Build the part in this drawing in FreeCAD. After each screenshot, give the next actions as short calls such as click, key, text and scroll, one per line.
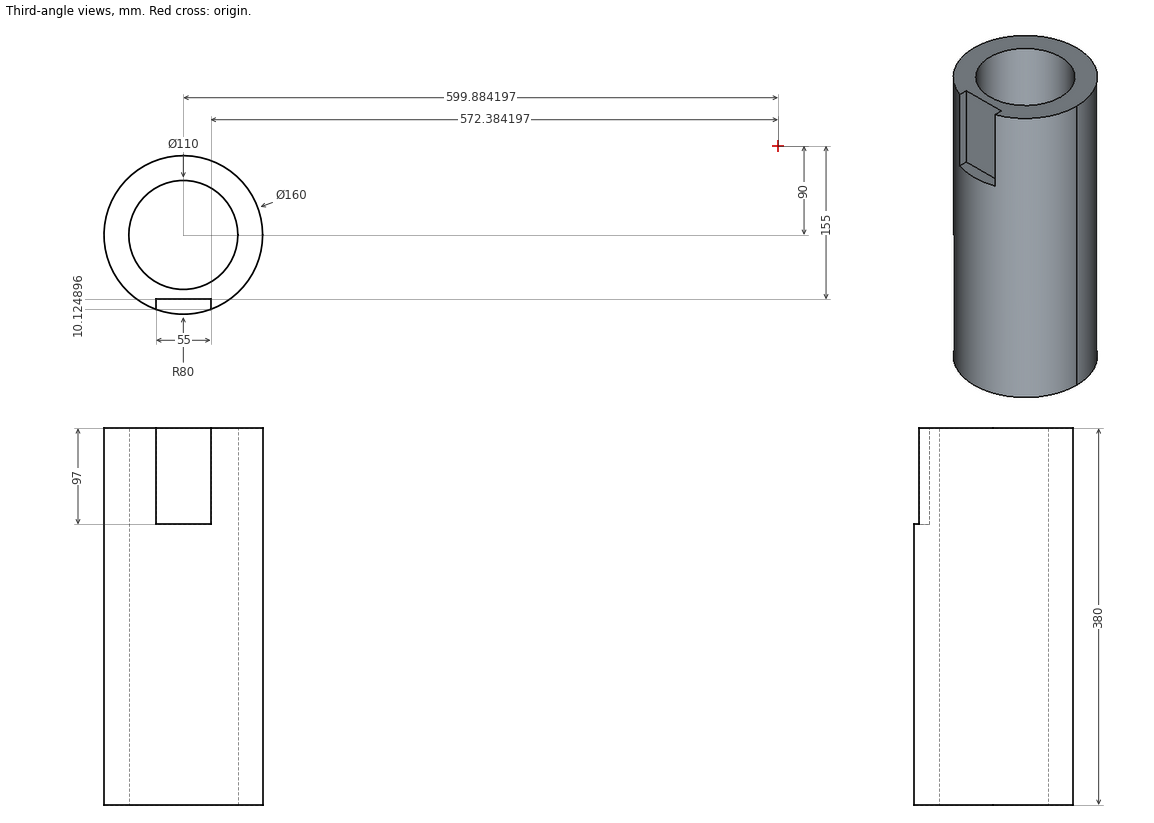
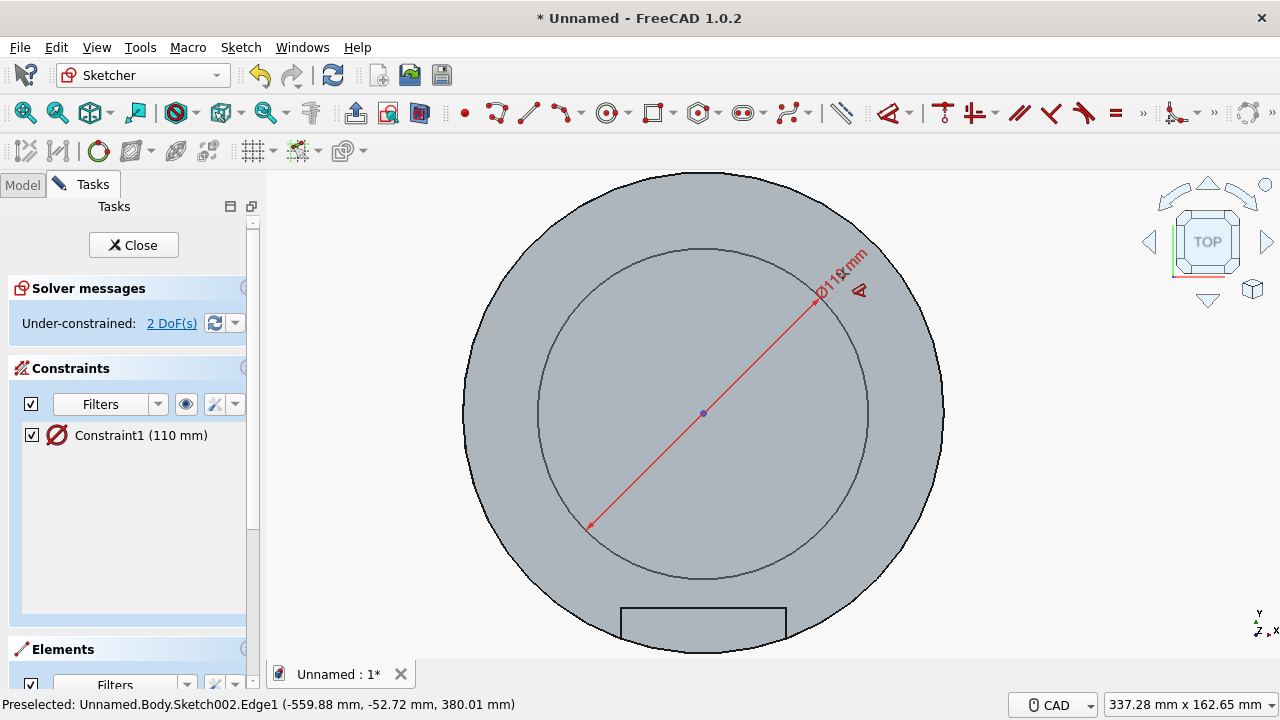
click(703, 414)
click(669, 306)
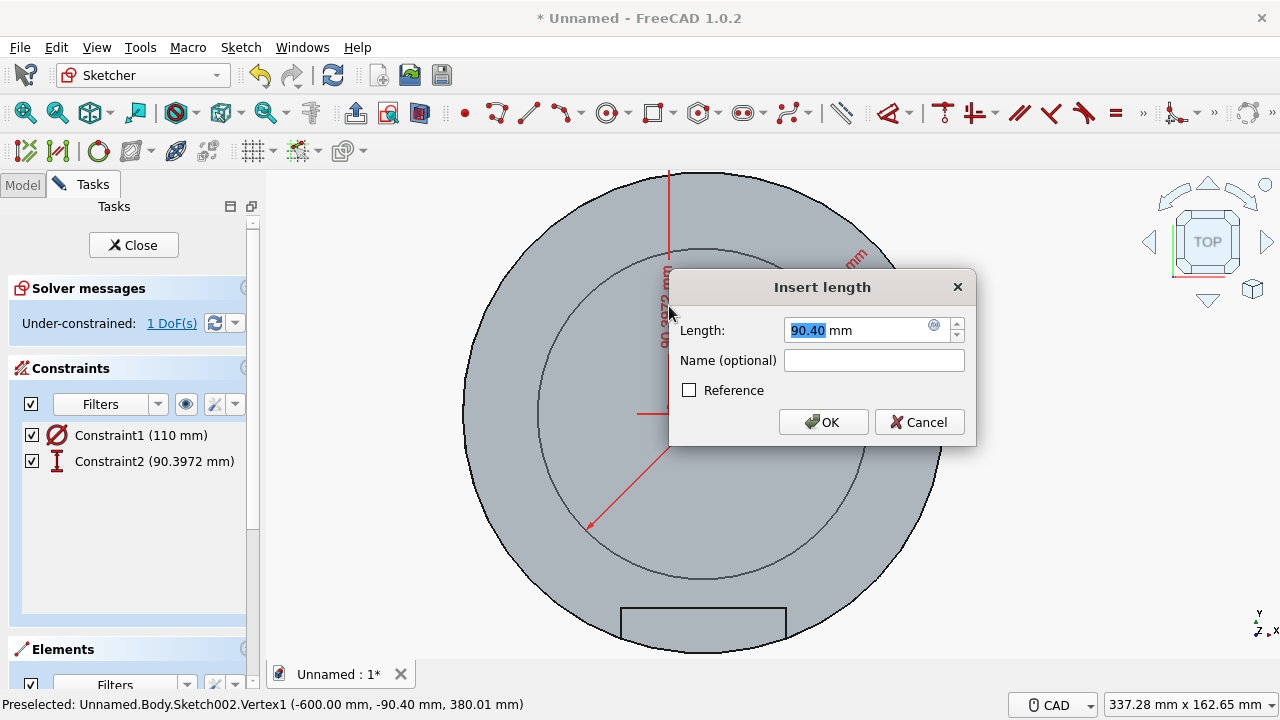
text(90)
key(Return)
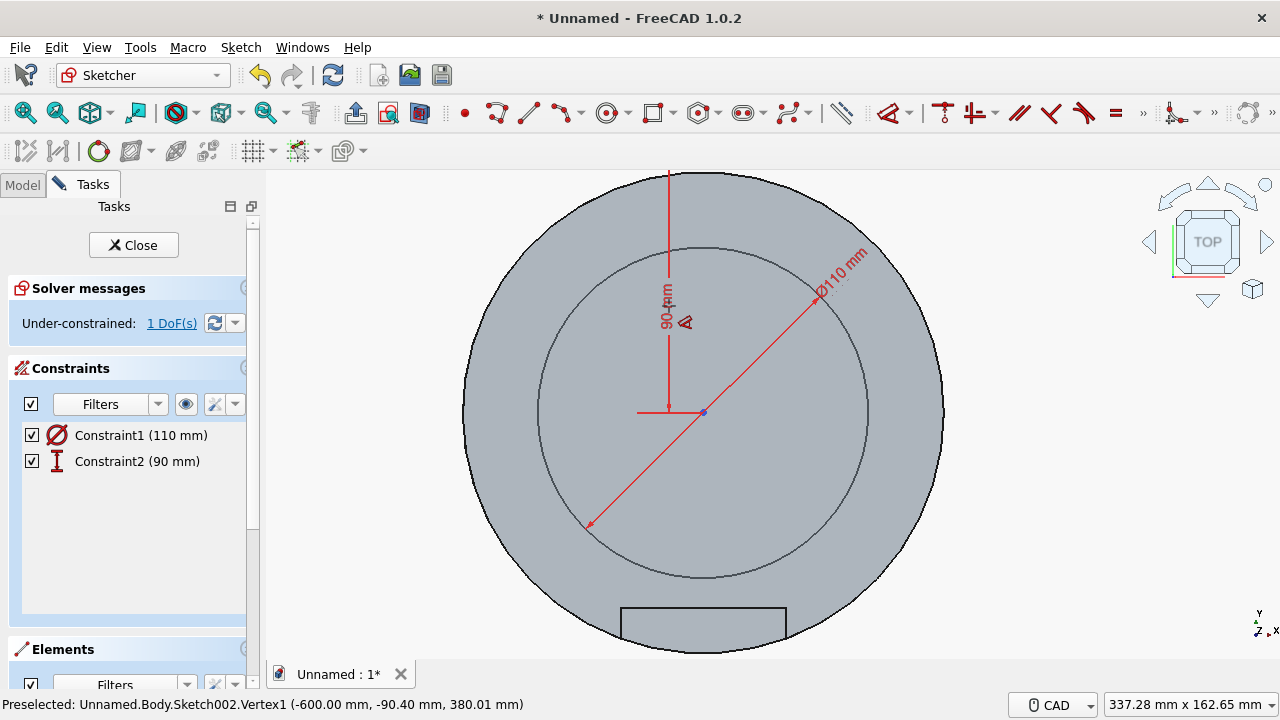
click(703, 413)
click(909, 447)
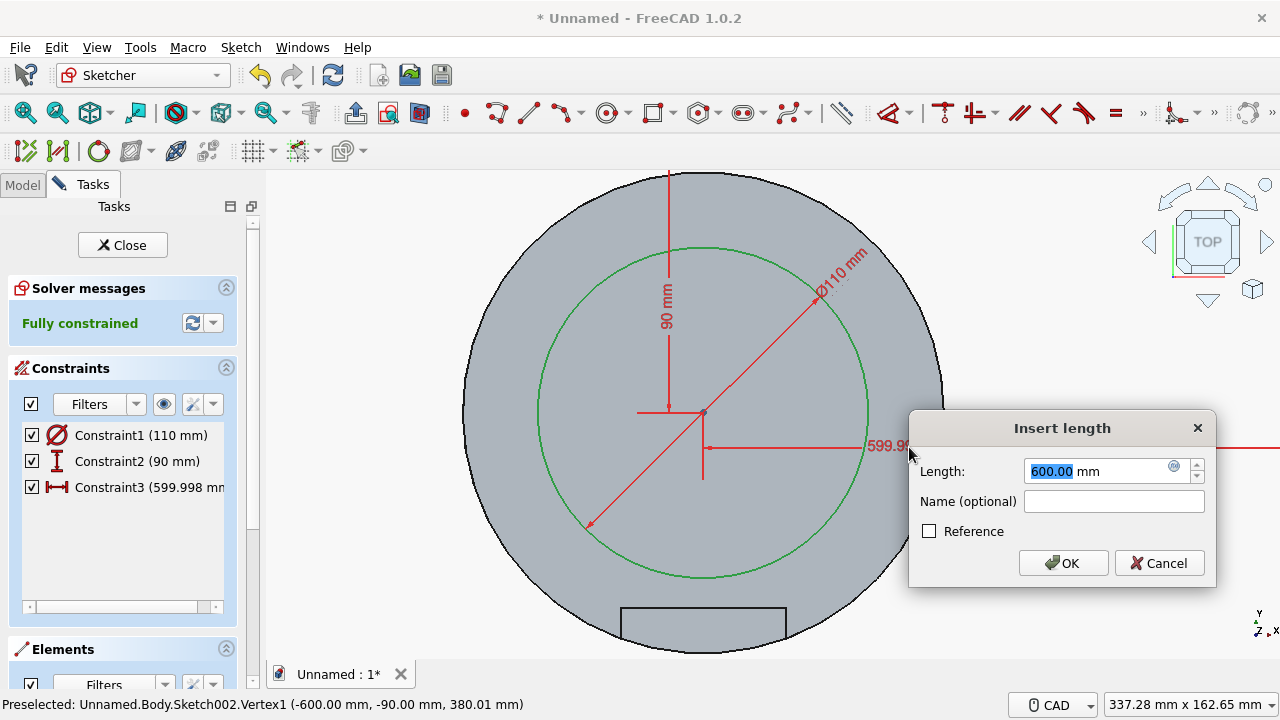
text(599.884197)
key(Return)
key(Escape)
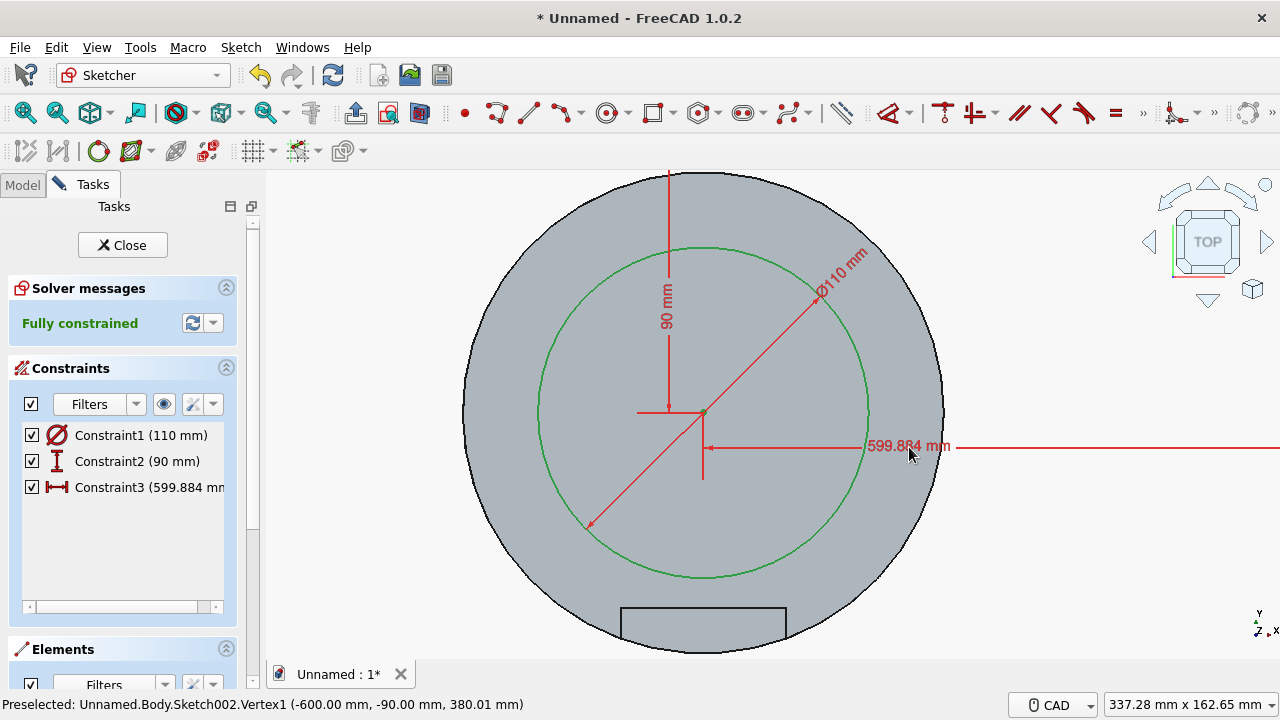
click(123, 245)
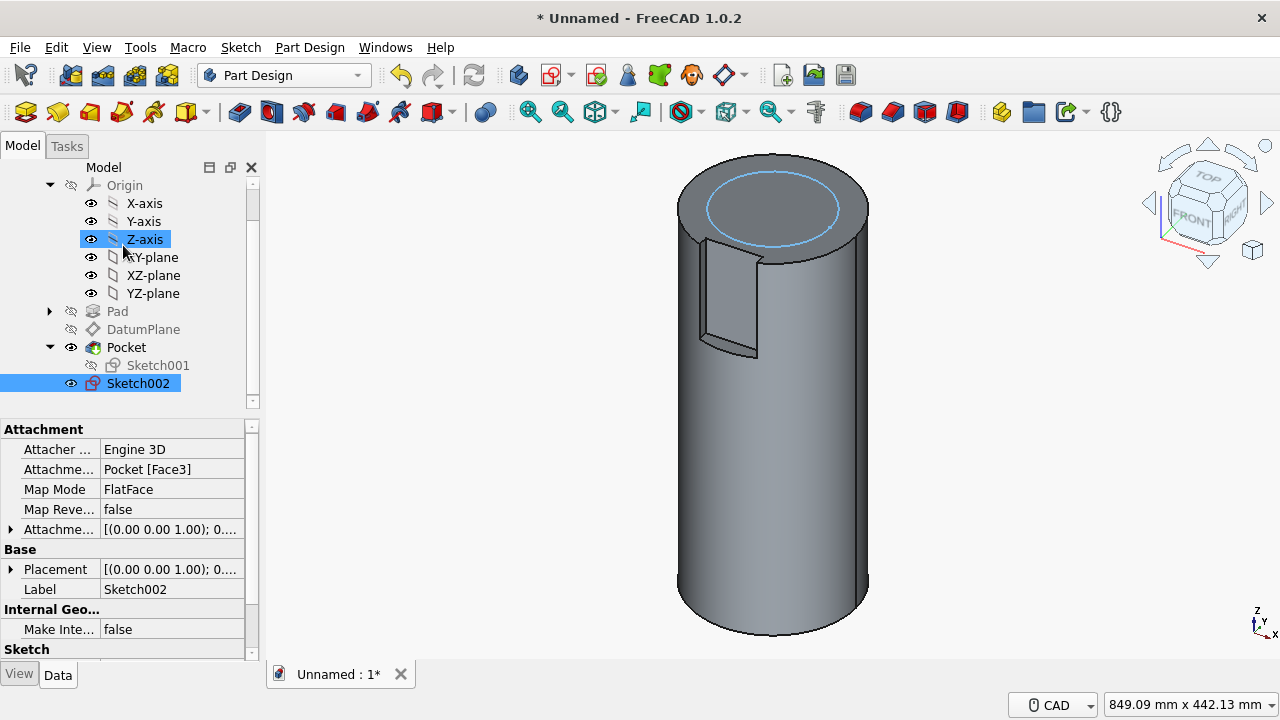
click(240, 112)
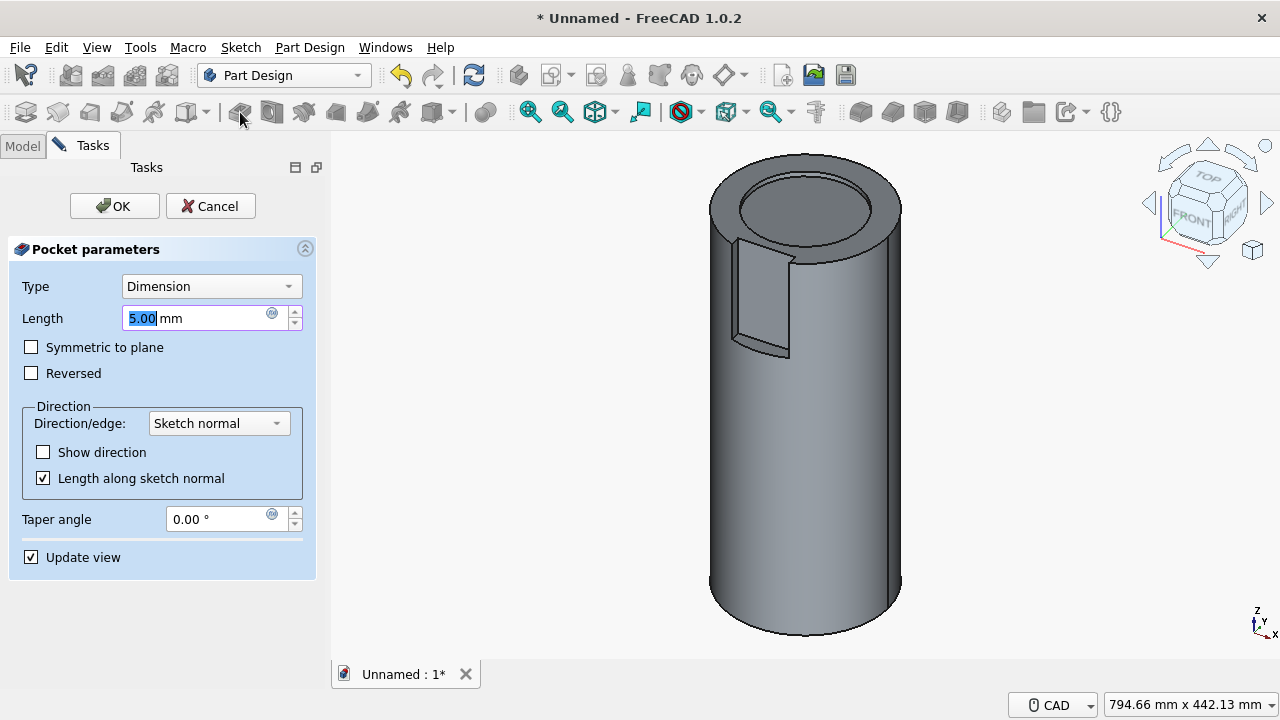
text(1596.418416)
key(Tab)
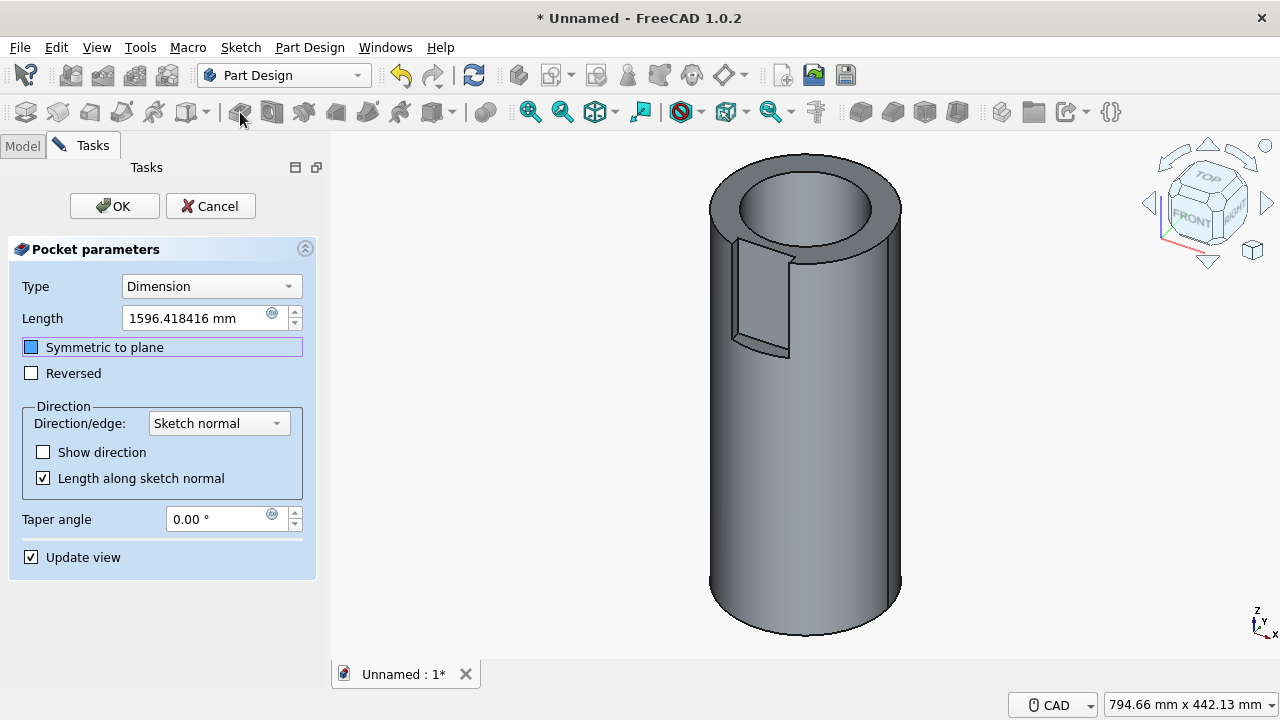
click(30, 347)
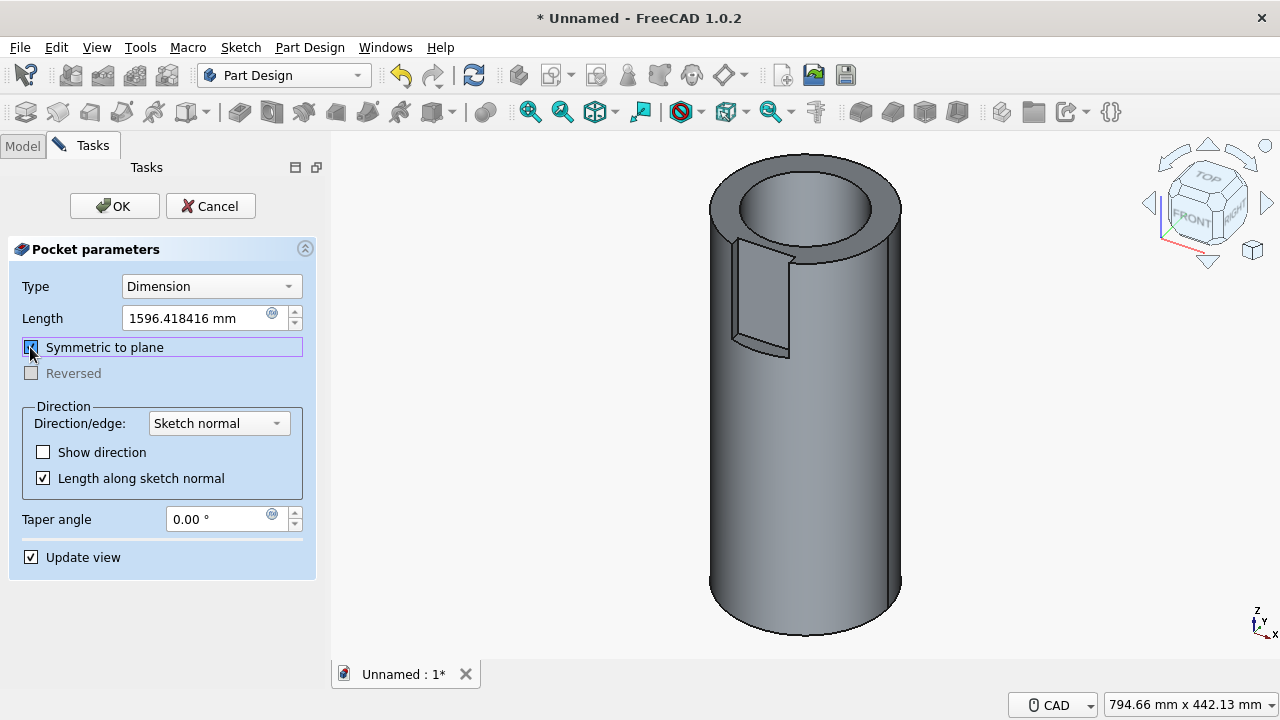
click(115, 206)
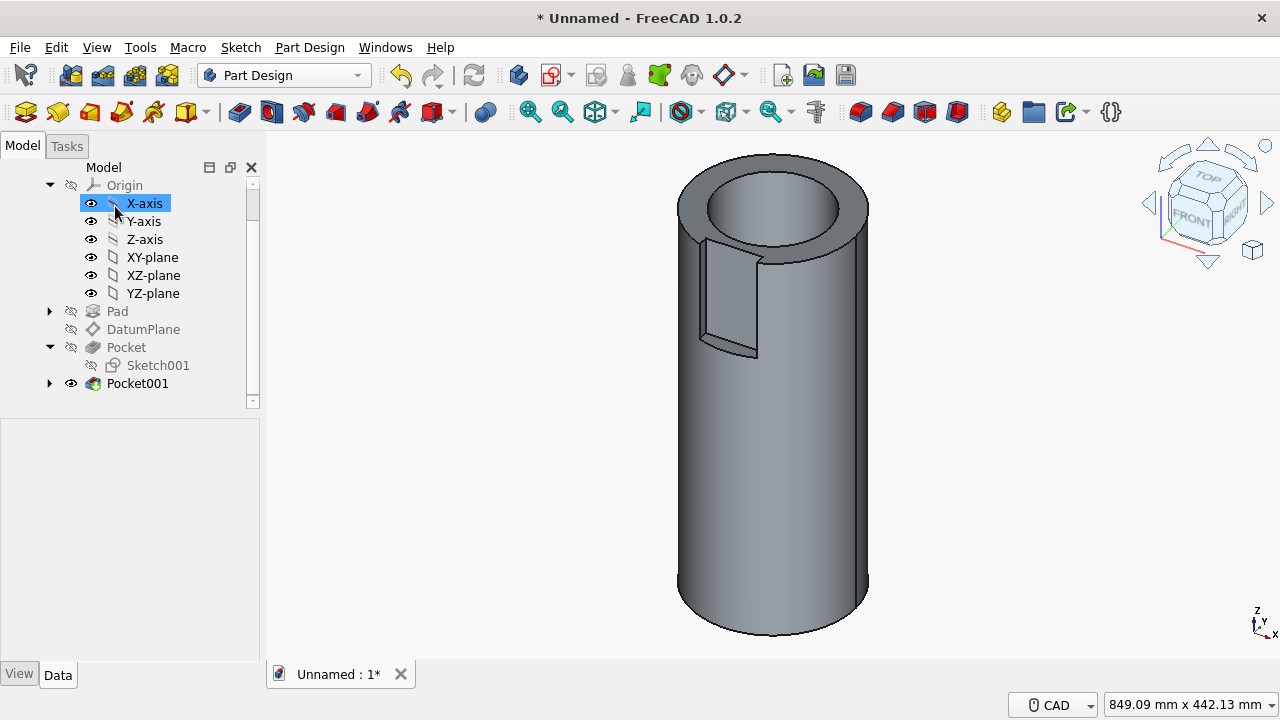
key(0)